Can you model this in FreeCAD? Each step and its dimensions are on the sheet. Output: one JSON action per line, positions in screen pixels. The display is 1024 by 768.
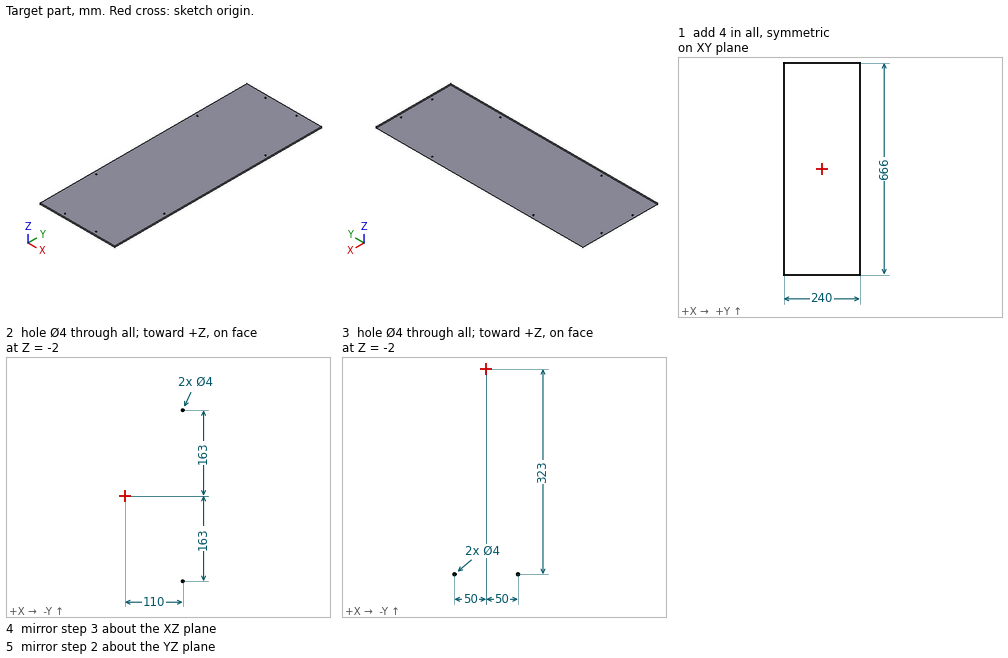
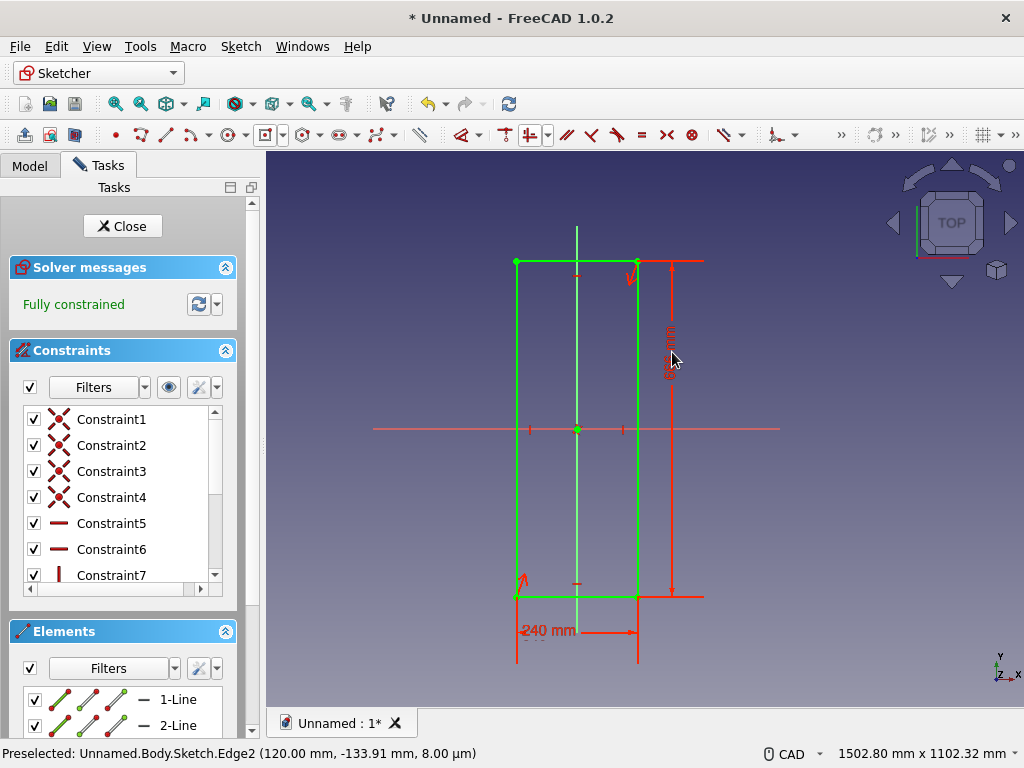
{"action": "left_click", "coordinate": [123, 226]}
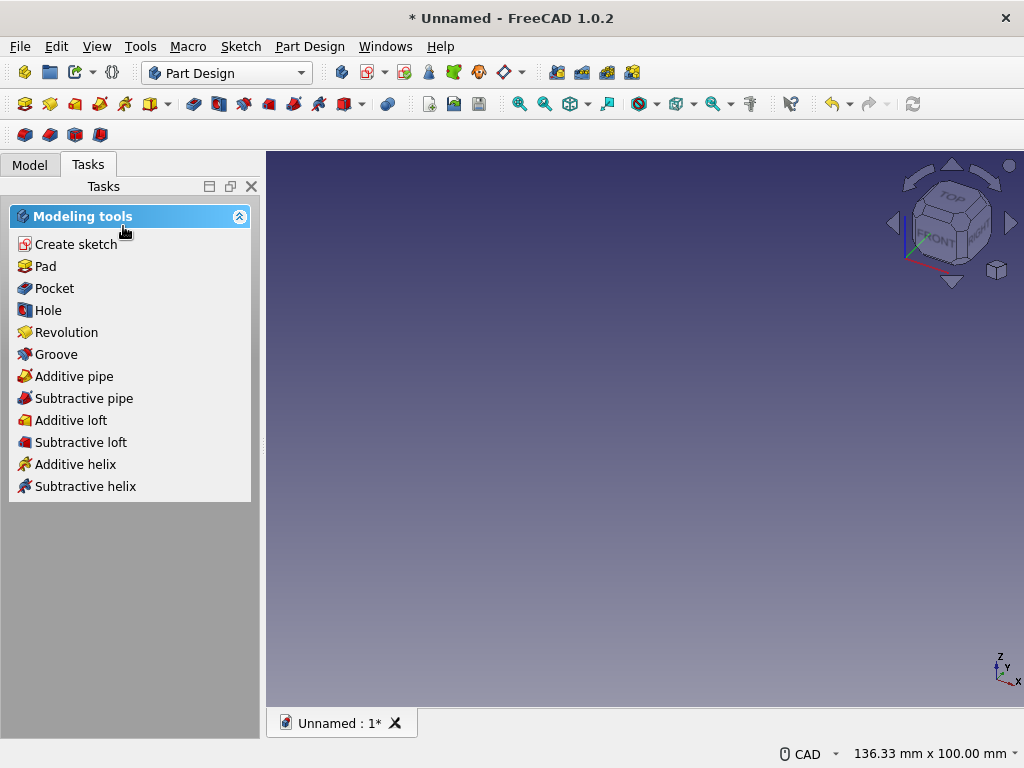
{"action": "left_click", "coordinate": [25, 104]}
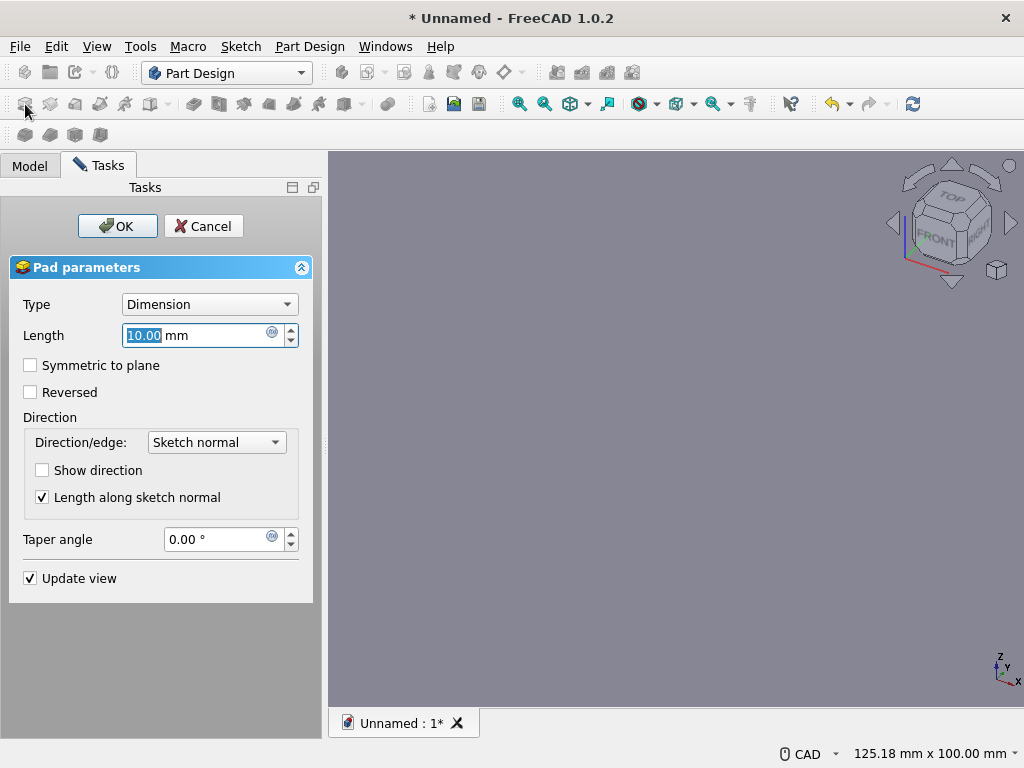
{"action": "type", "text": "4"}
{"action": "key", "text": "Tab"}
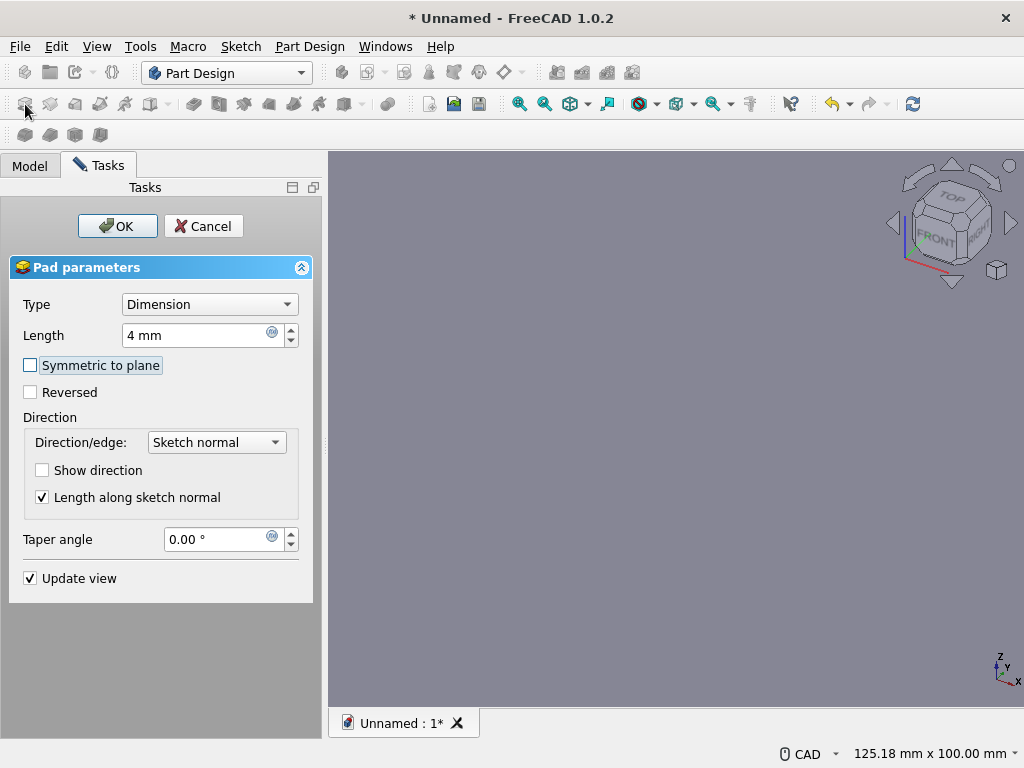
{"action": "left_click", "coordinate": [31, 365]}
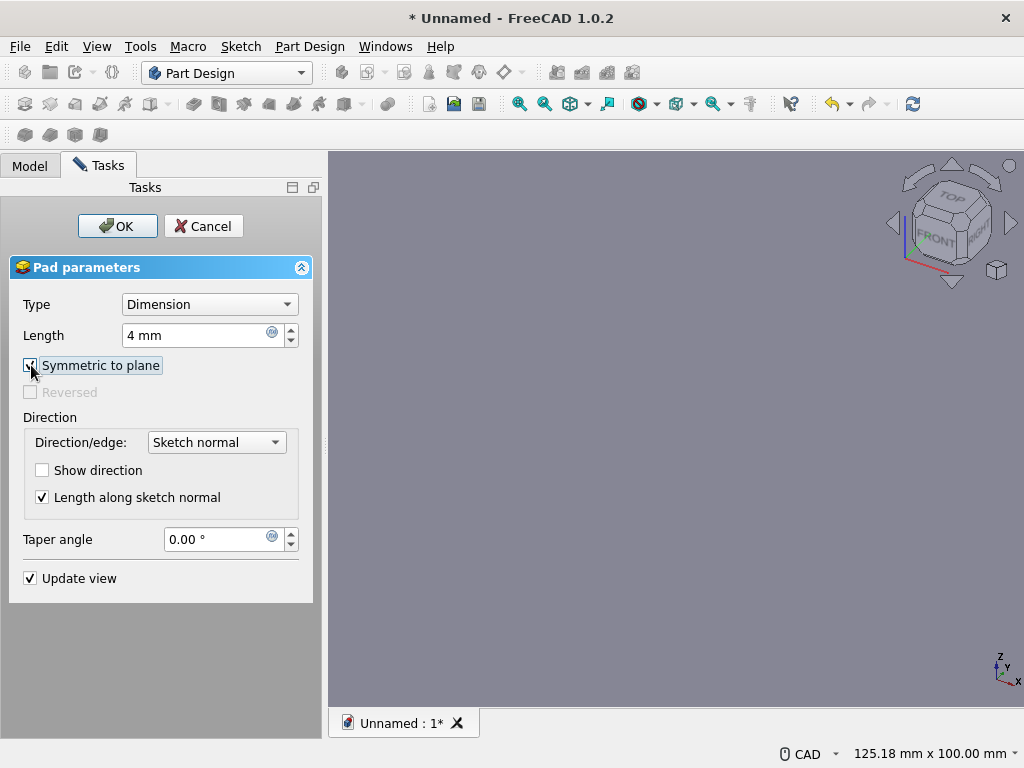
{"action": "left_click", "coordinate": [118, 226]}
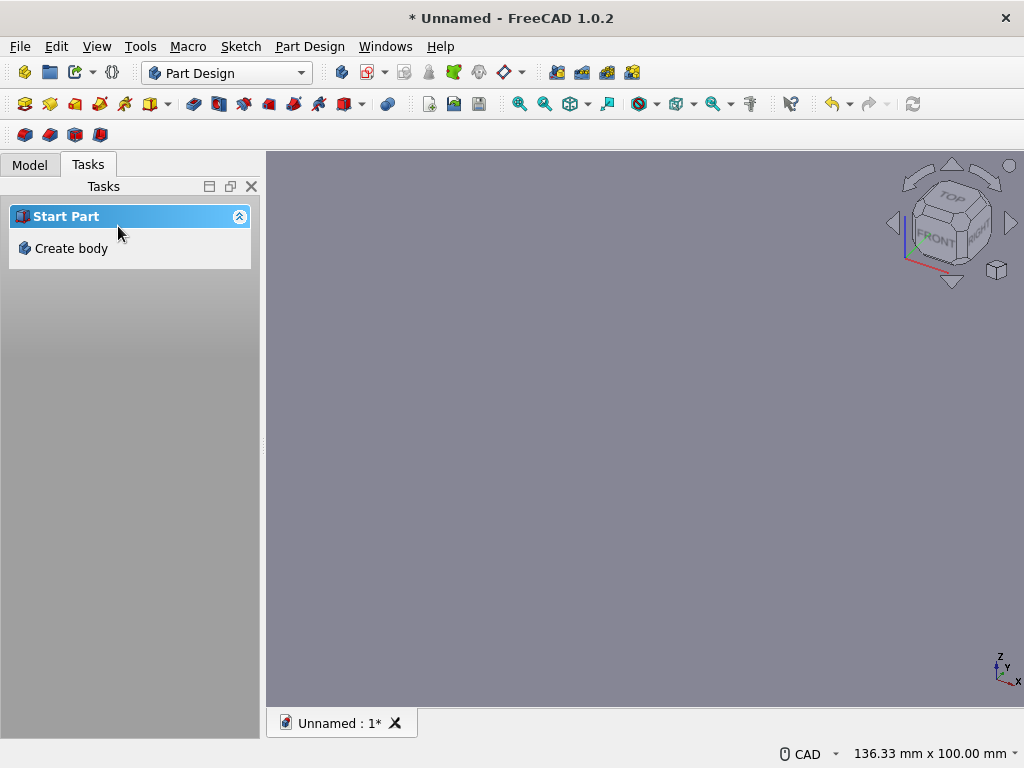
{"action": "left_click", "coordinate": [520, 104]}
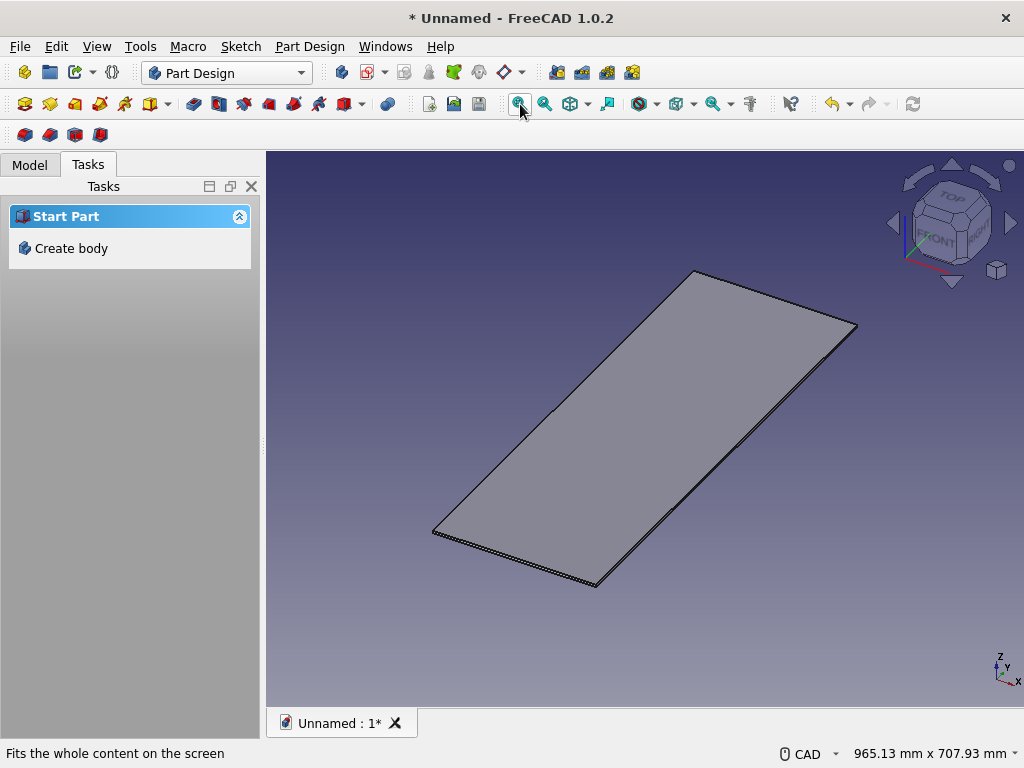
{"action": "key", "text": "5"}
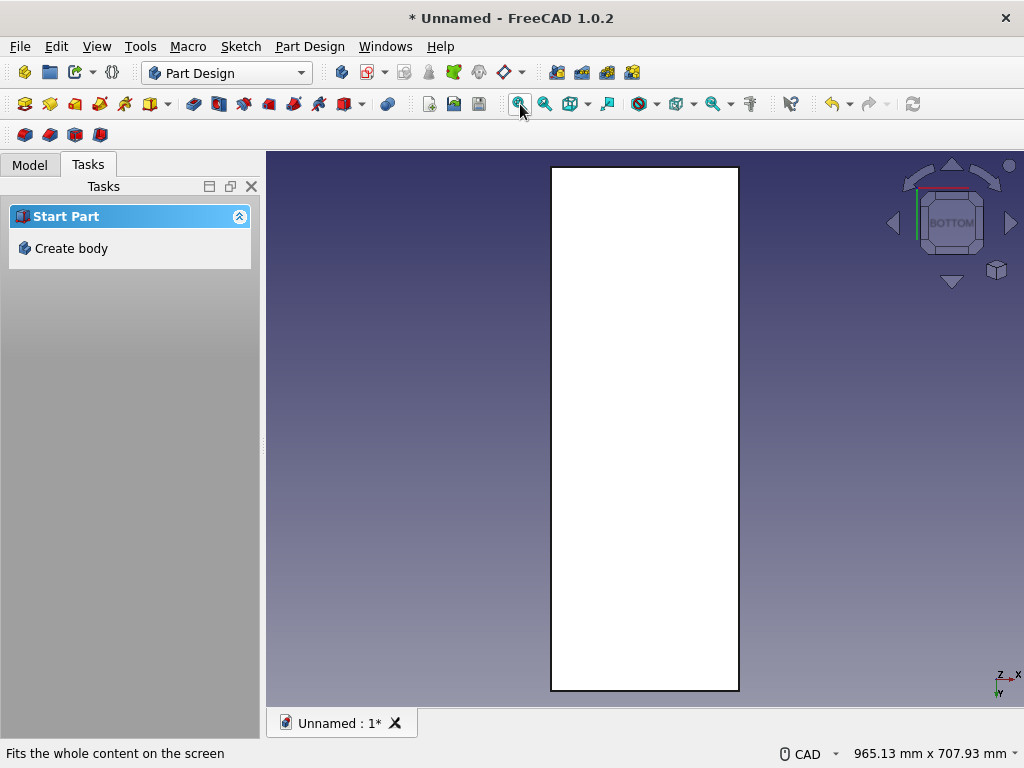
{"action": "left_click", "coordinate": [645, 577]}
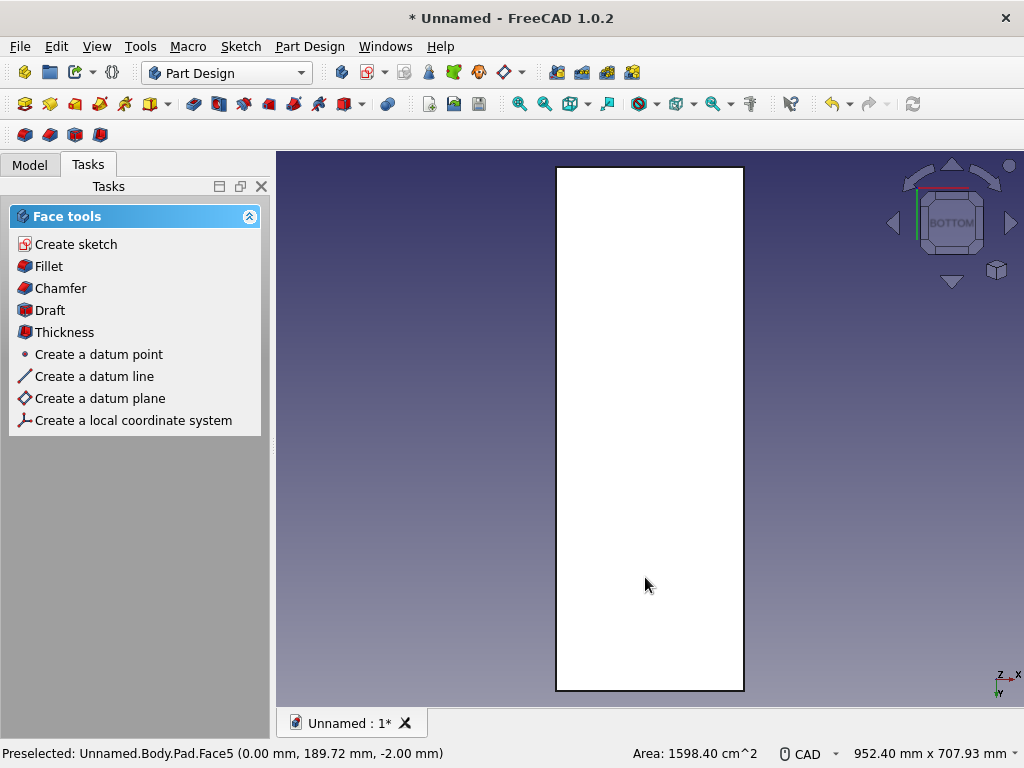
{"action": "left_click", "coordinate": [366, 72]}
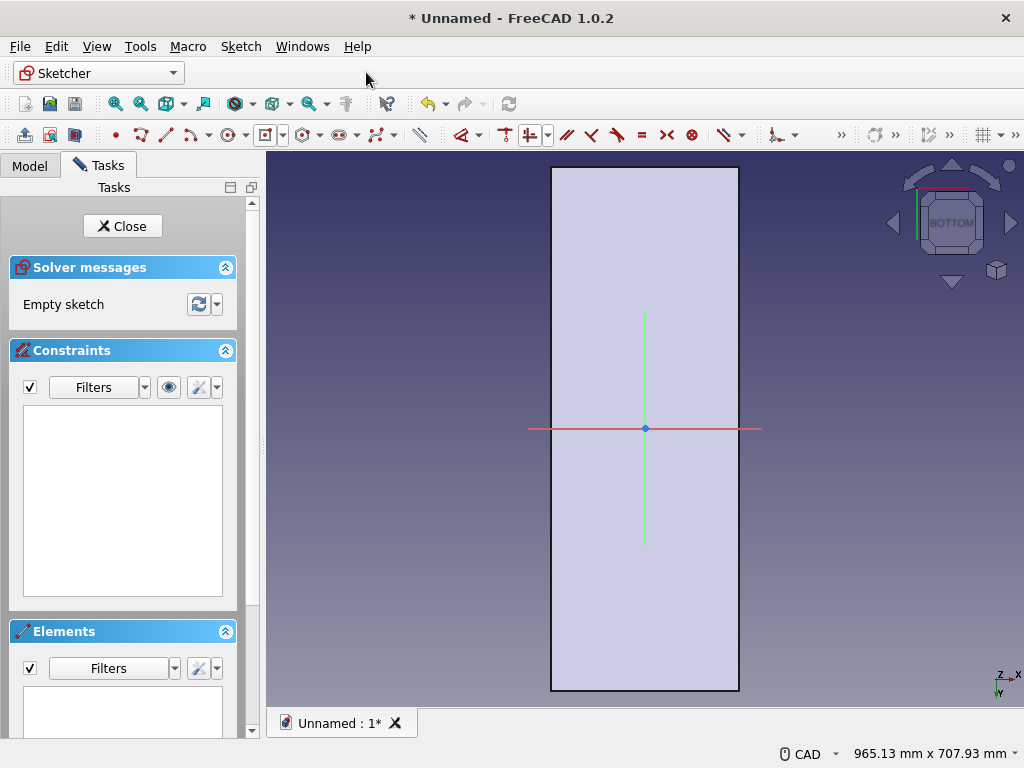
{"action": "scroll", "coordinate": [859, 429], "scroll_direction": "up", "scroll_amount": 2}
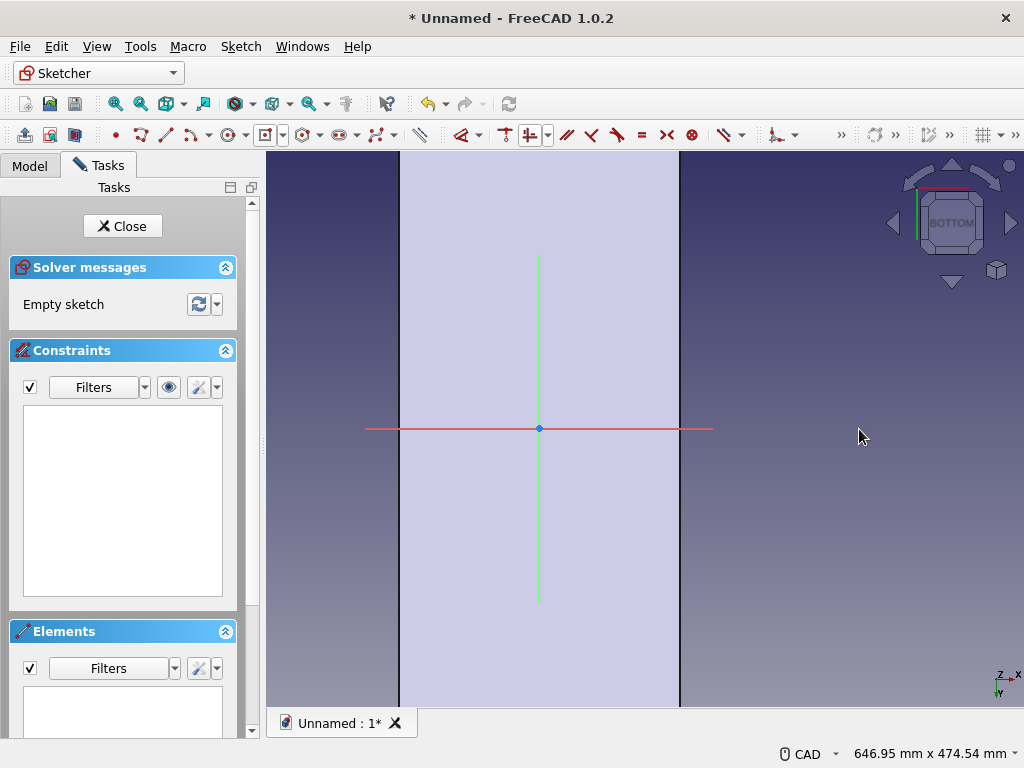
{"action": "left_click", "coordinate": [228, 136]}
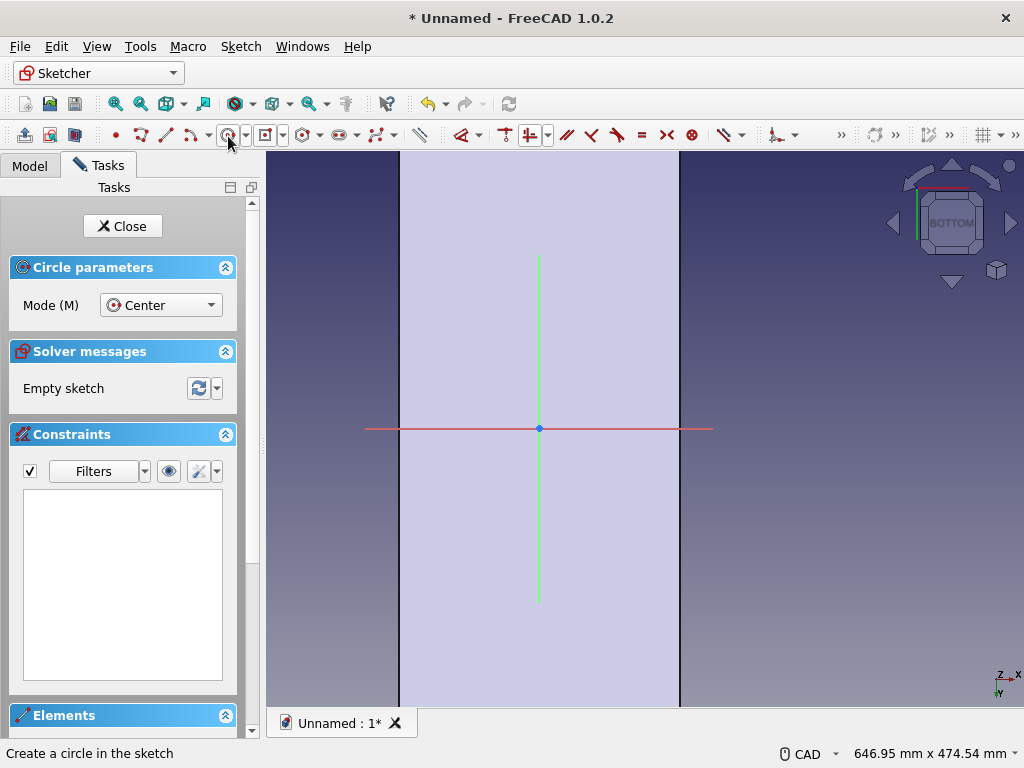
{"action": "scroll", "coordinate": [668, 620], "scroll_direction": "up", "scroll_amount": 12}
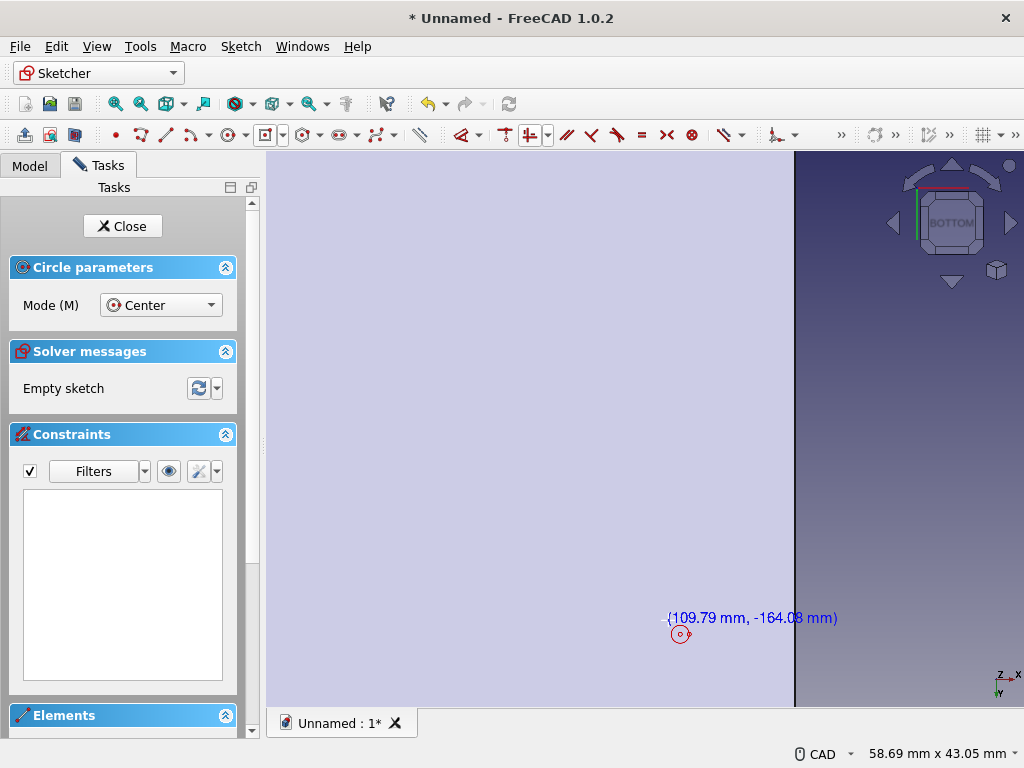
{"action": "scroll", "coordinate": [637, 621], "scroll_direction": "down", "scroll_amount": 12}